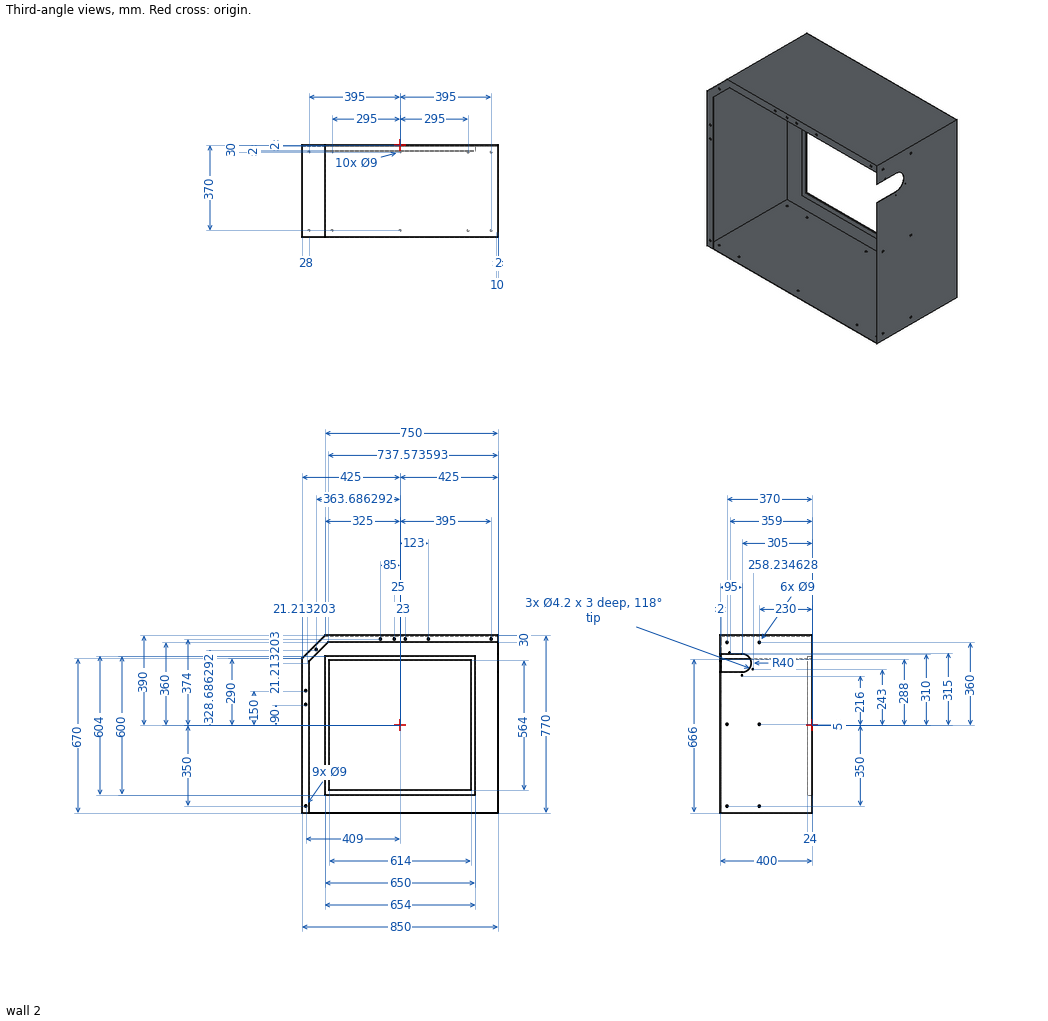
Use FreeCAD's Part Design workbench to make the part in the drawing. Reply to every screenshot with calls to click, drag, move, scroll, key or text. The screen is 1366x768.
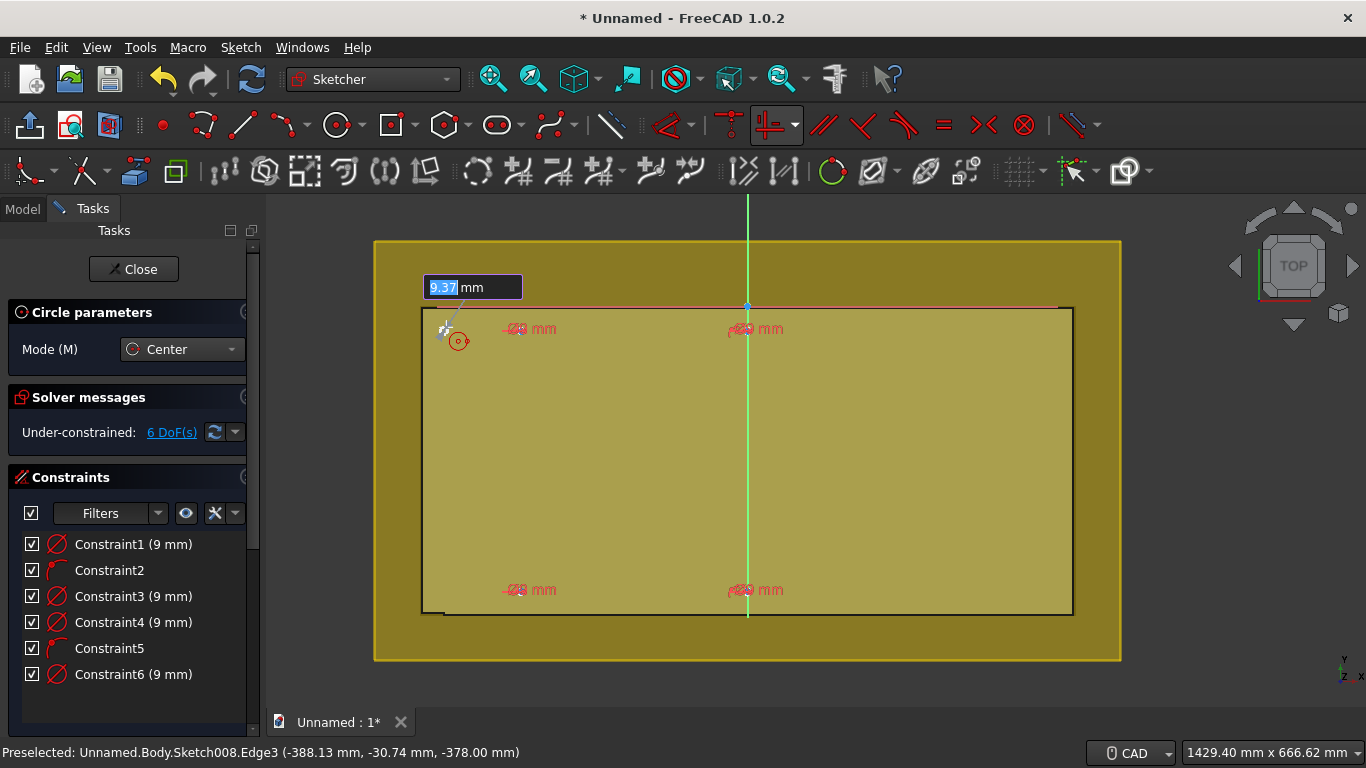
text(9)
key(Return)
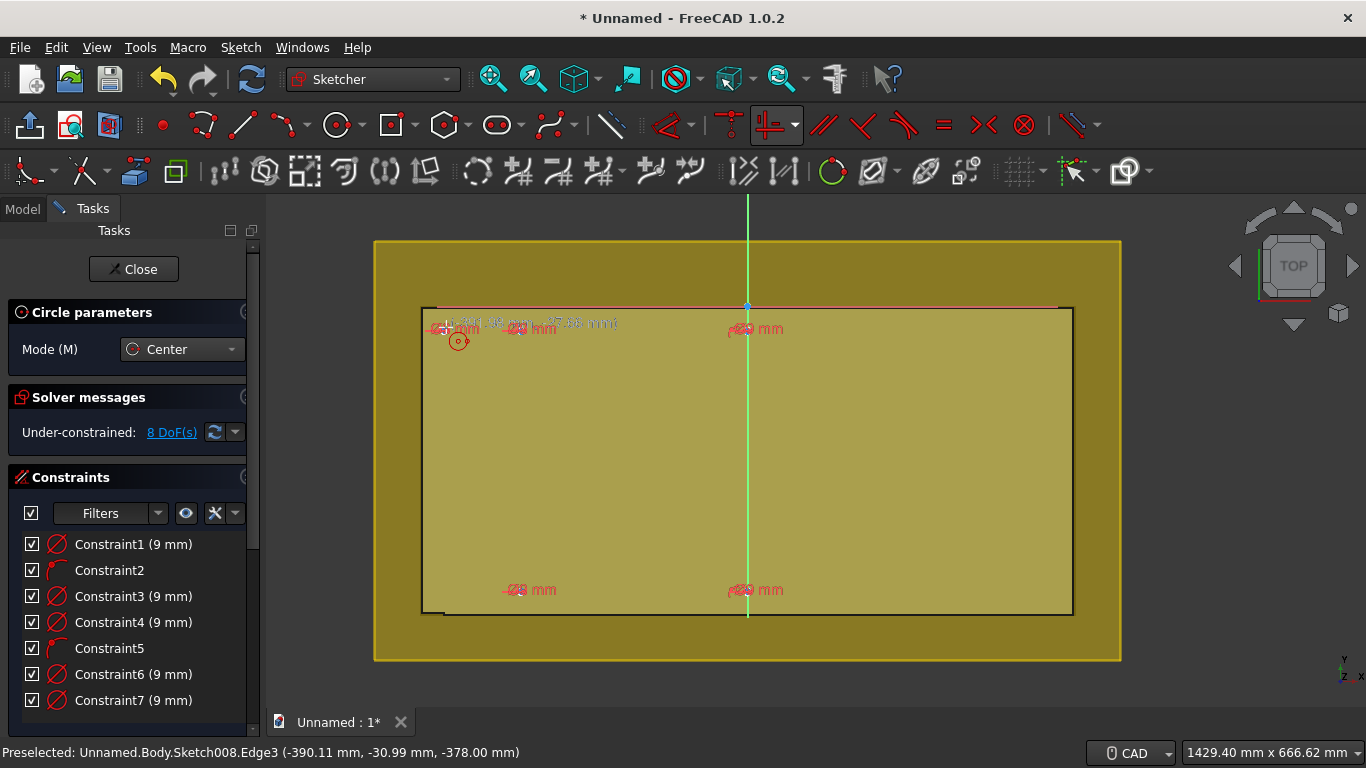
scroll(444, 591, up, 10)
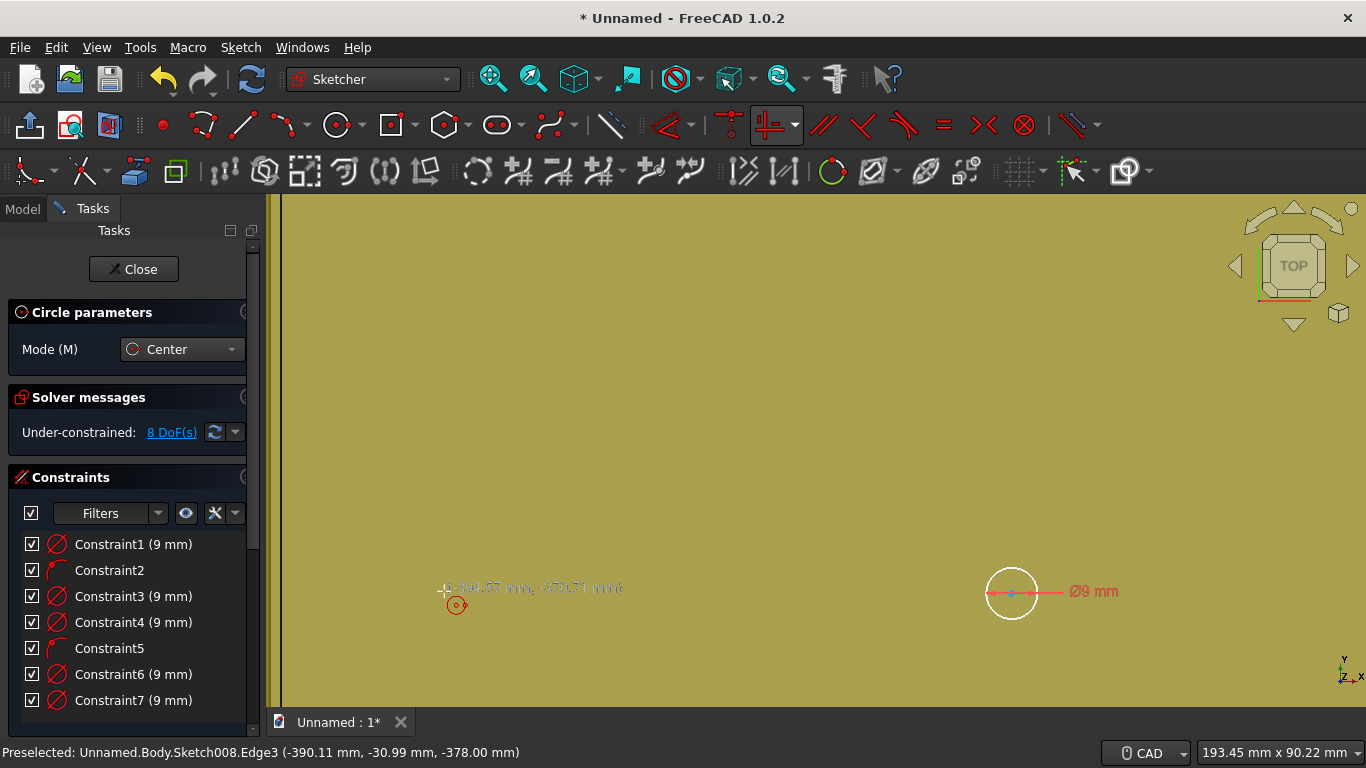
scroll(444, 591, down, 10)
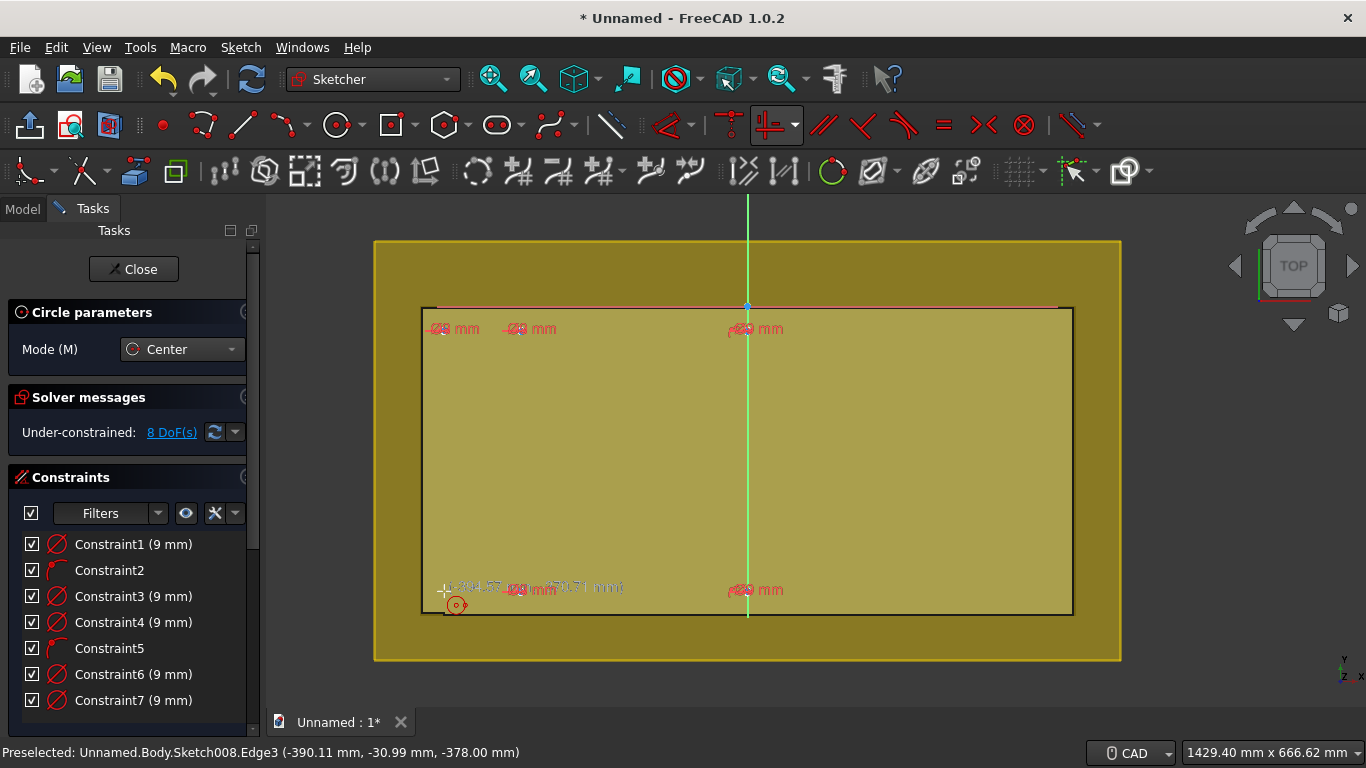
click(444, 591)
move(446, 589)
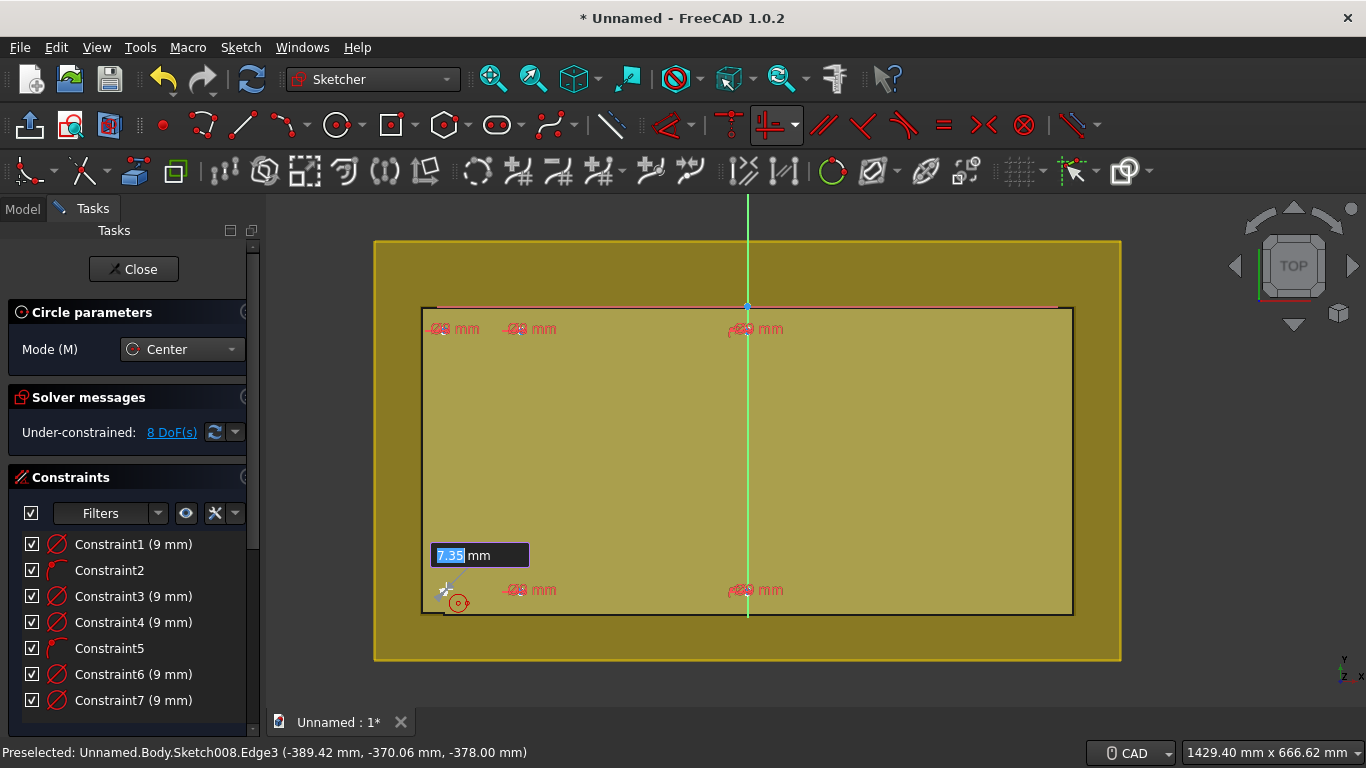
text(9)
key(Return)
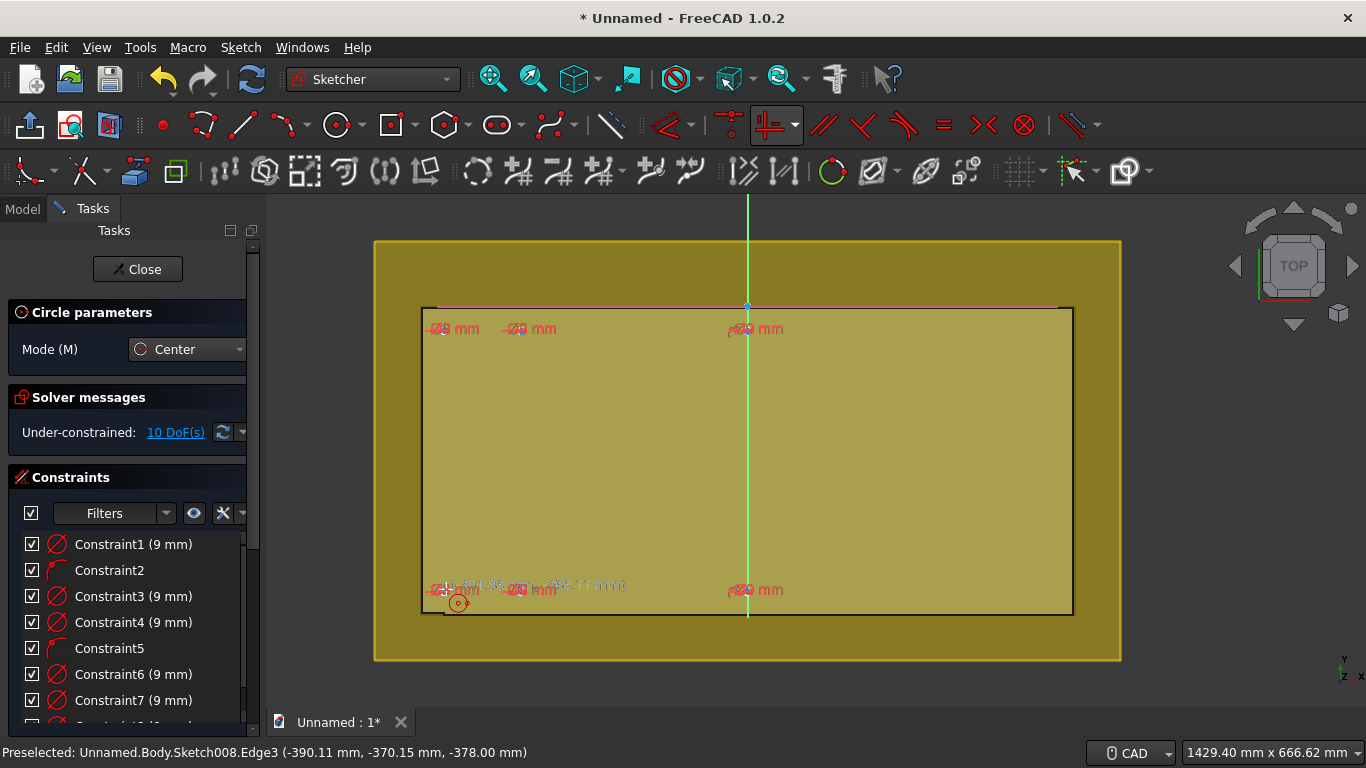
scroll(975, 330, up, 10)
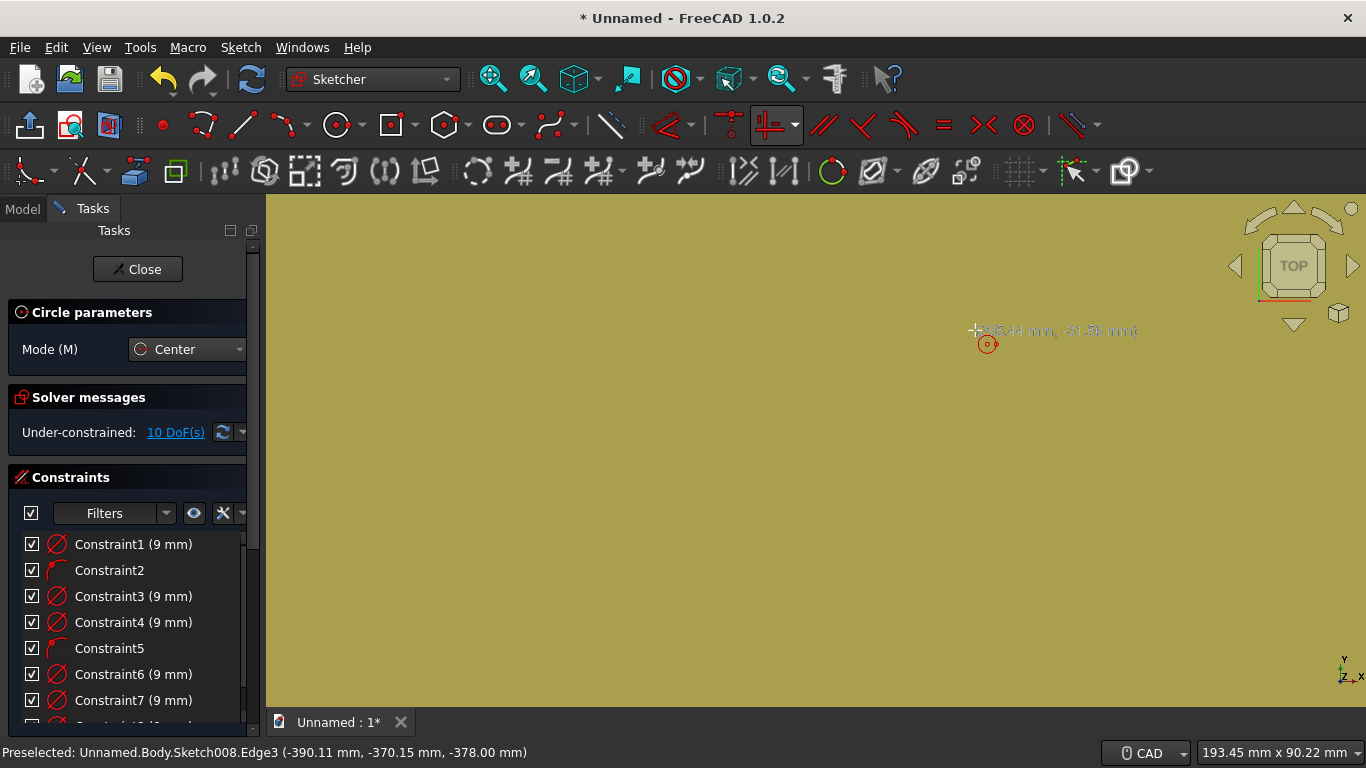
scroll(975, 330, down, 10)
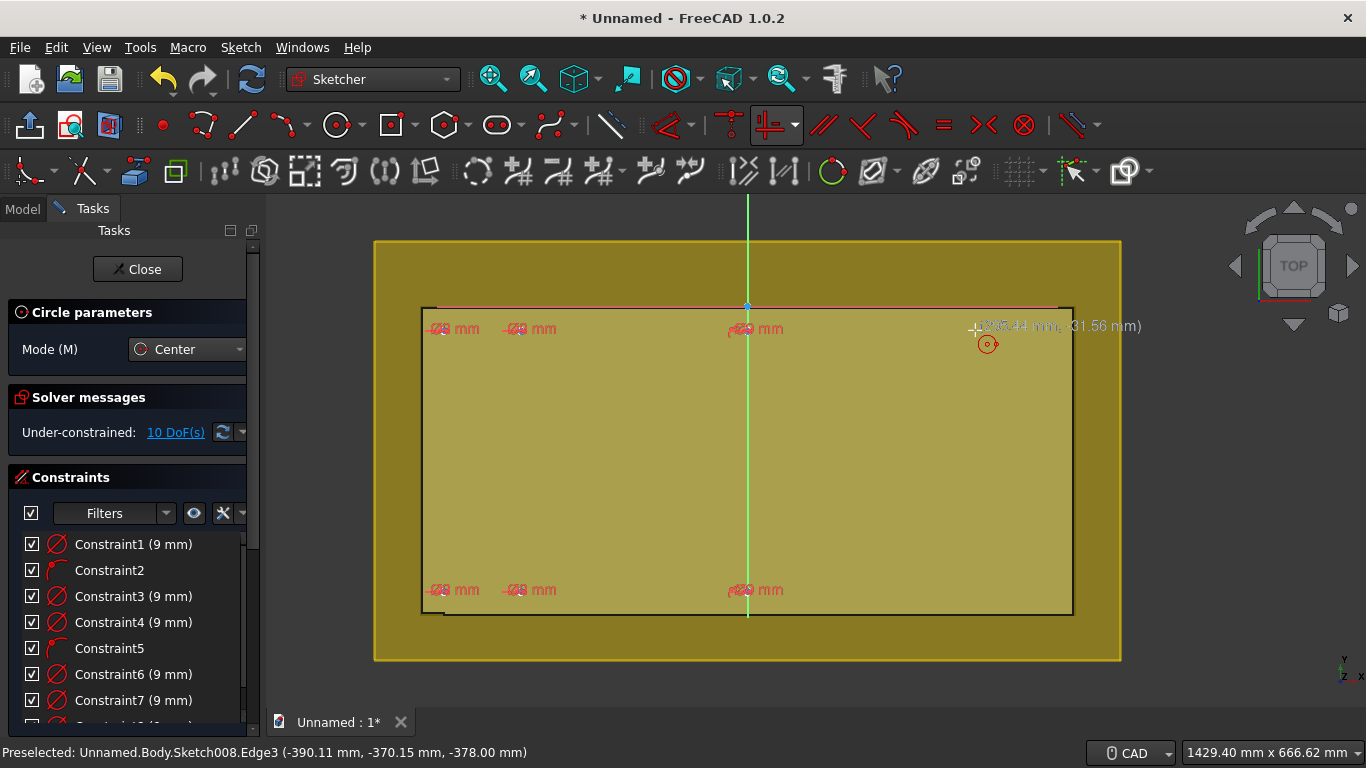
click(975, 330)
move(977, 327)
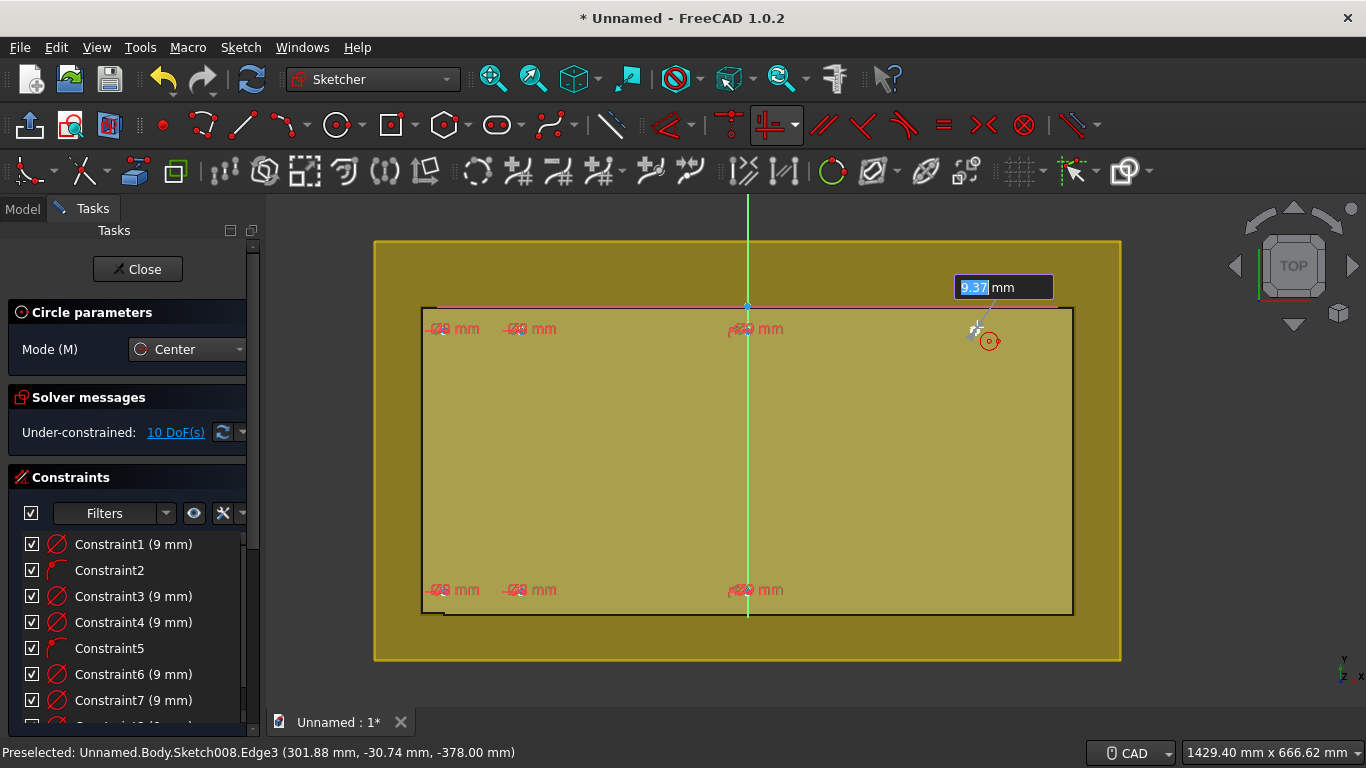
text(9)
key(Return)